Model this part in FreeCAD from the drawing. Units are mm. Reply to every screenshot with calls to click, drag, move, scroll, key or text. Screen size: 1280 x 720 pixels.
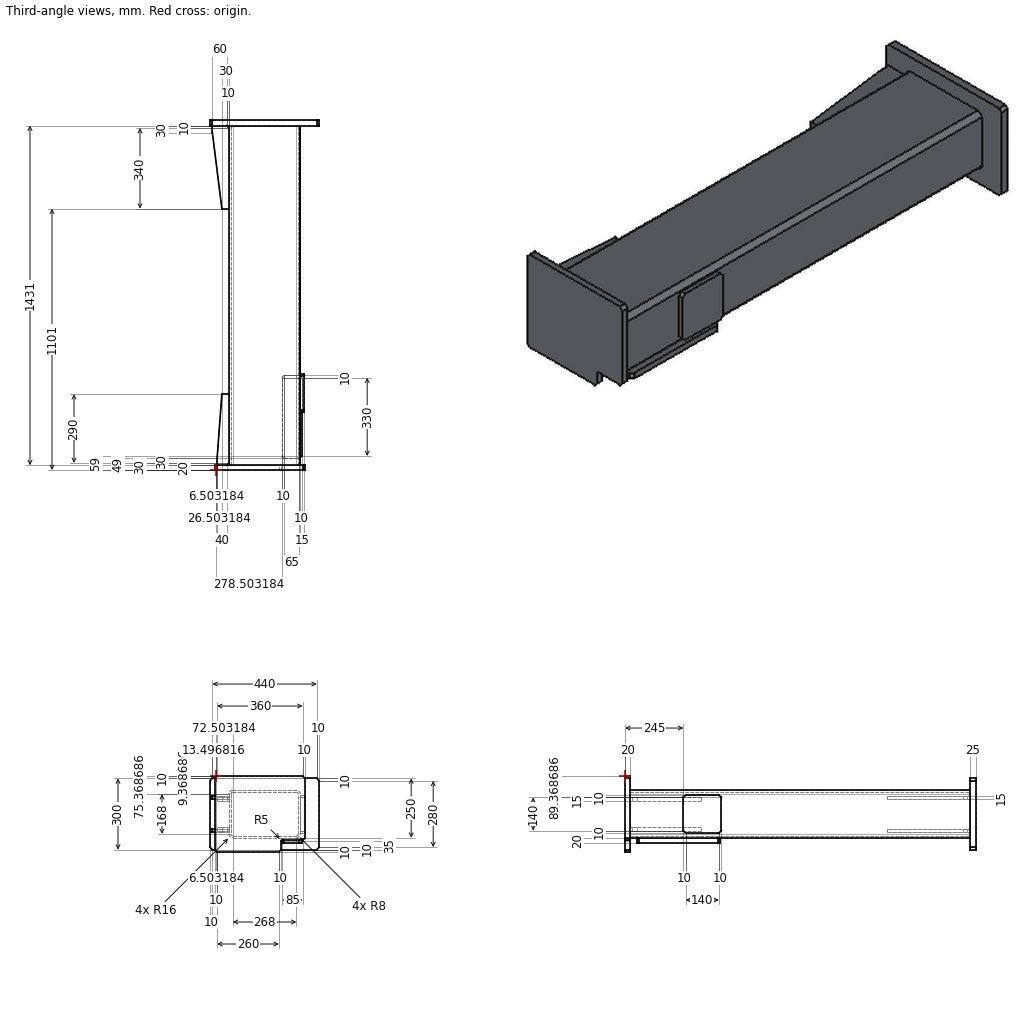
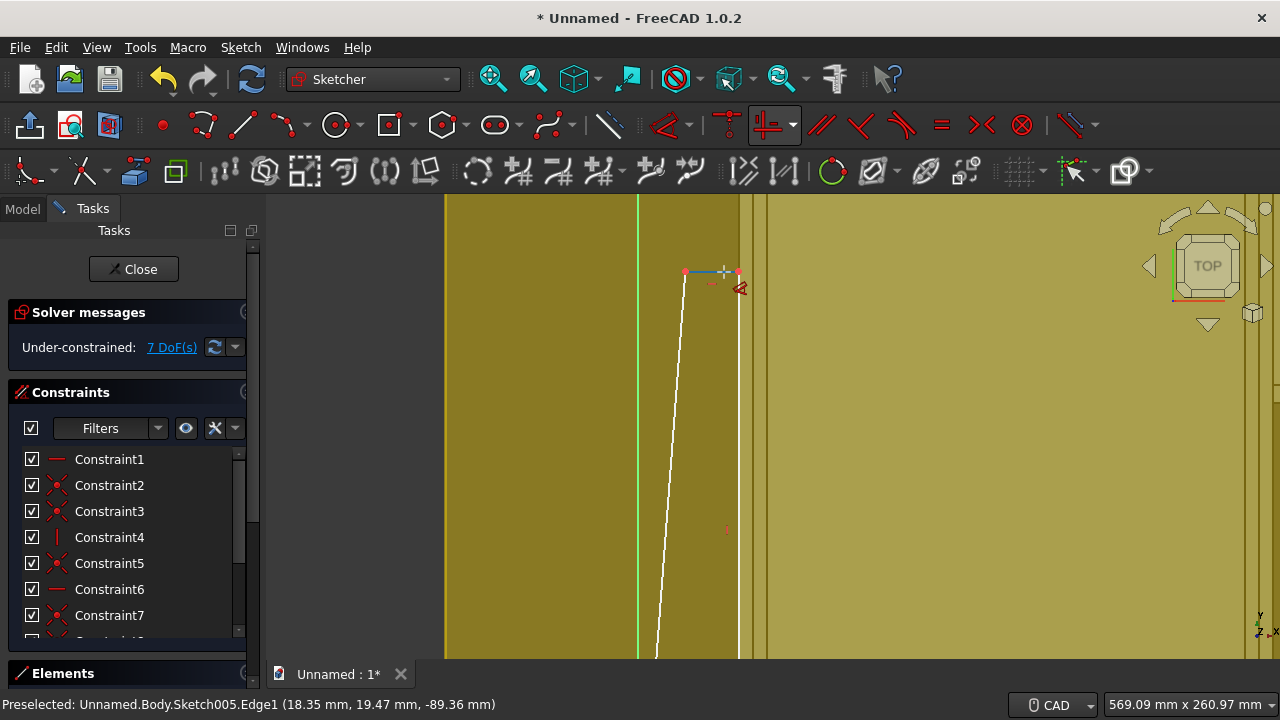
click(723, 272)
click(712, 238)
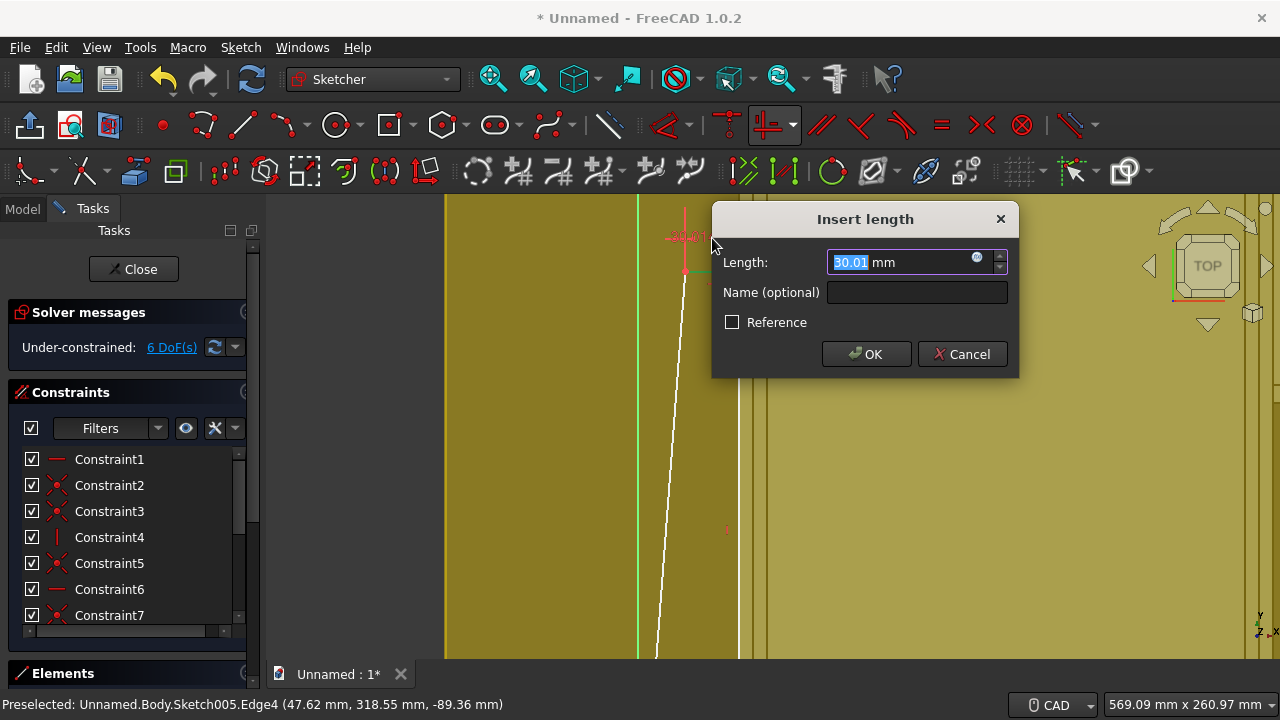
text(30)
key(Return)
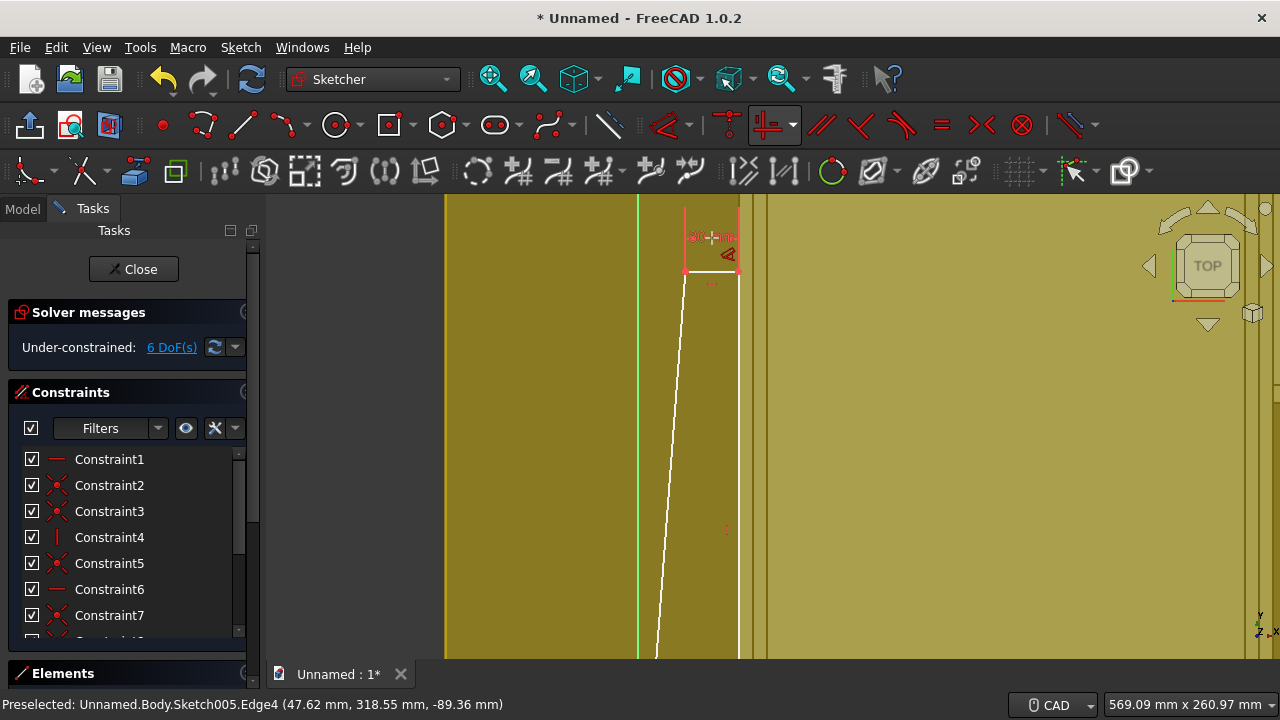
scroll(724, 271, down, 3)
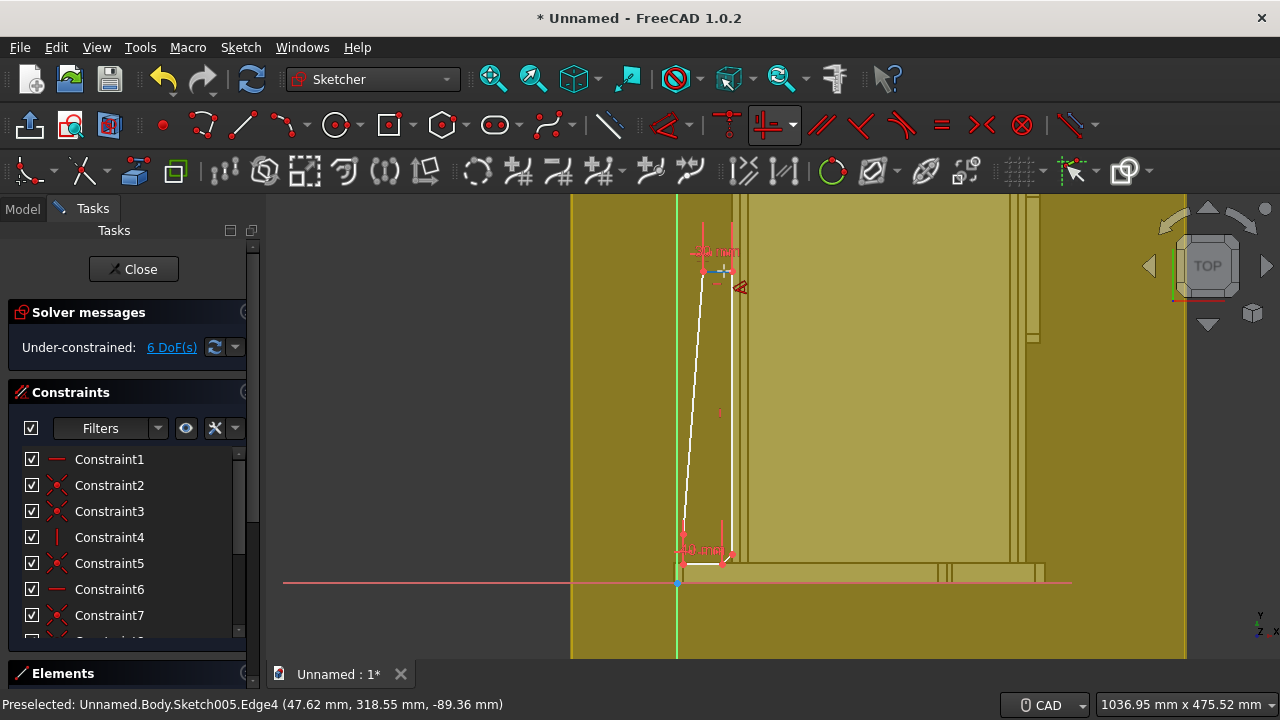
scroll(683, 543, up, 5)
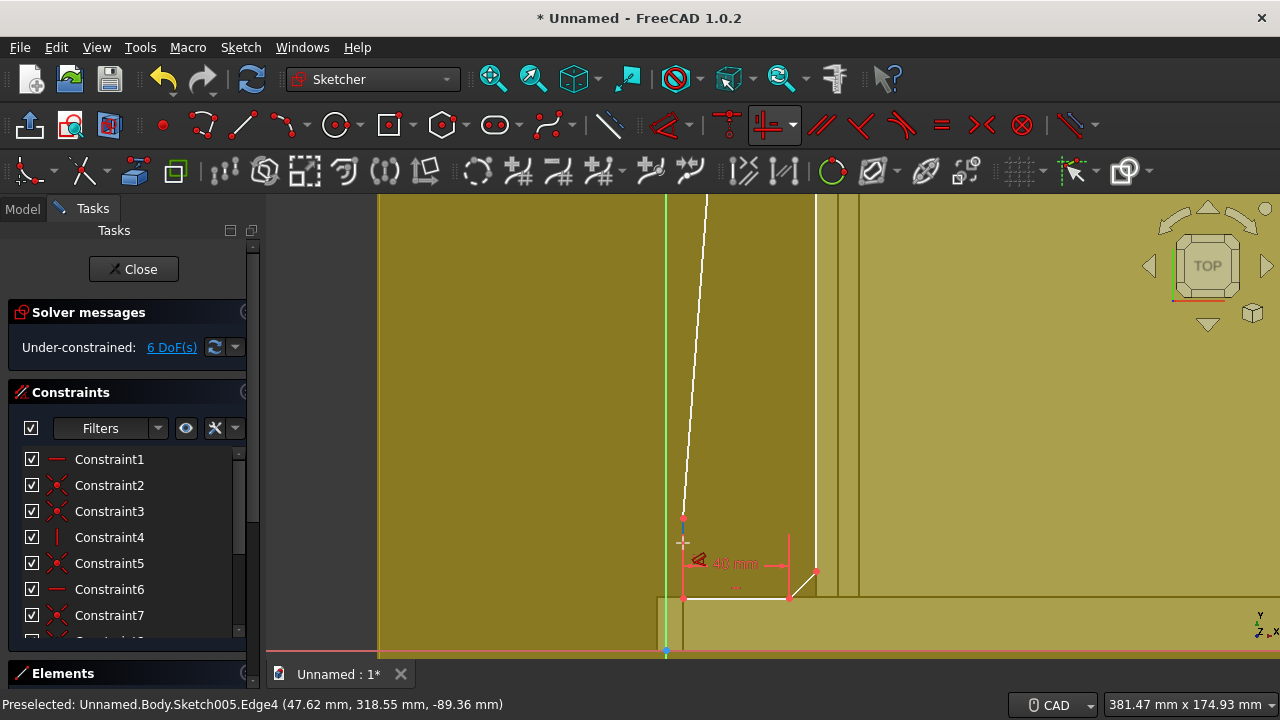
click(683, 543)
click(649, 559)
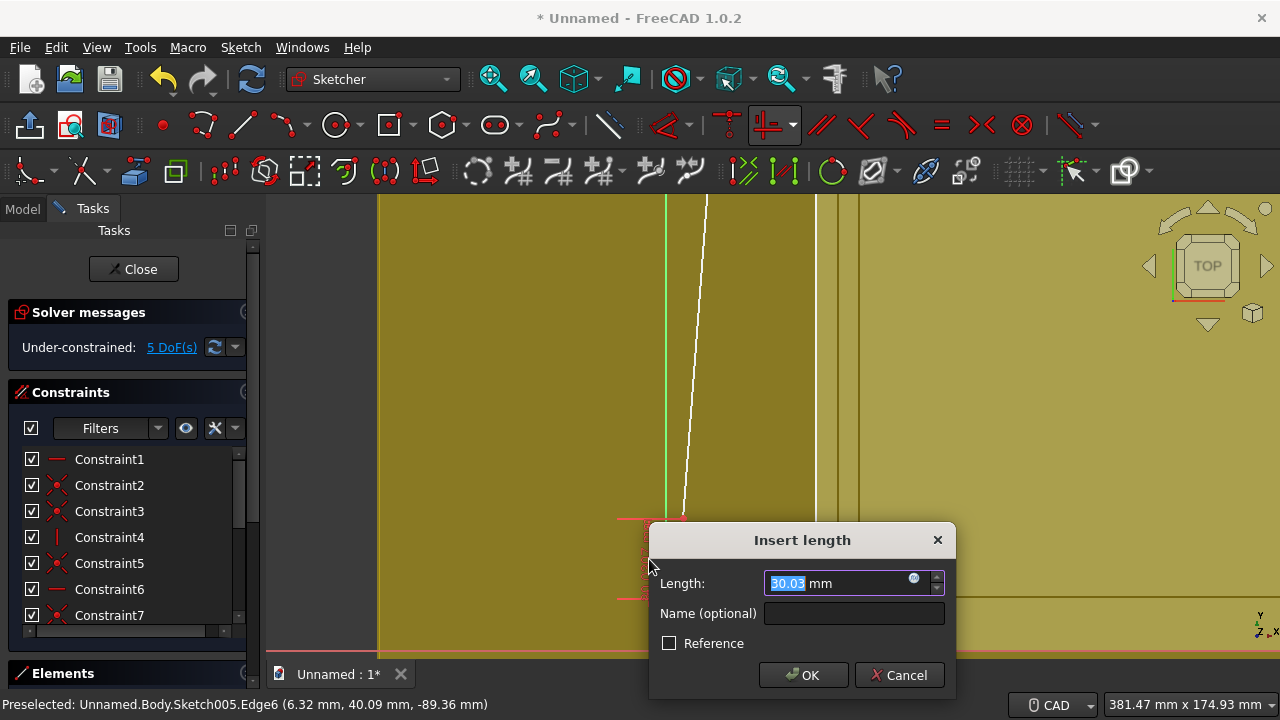
text(30)
key(Return)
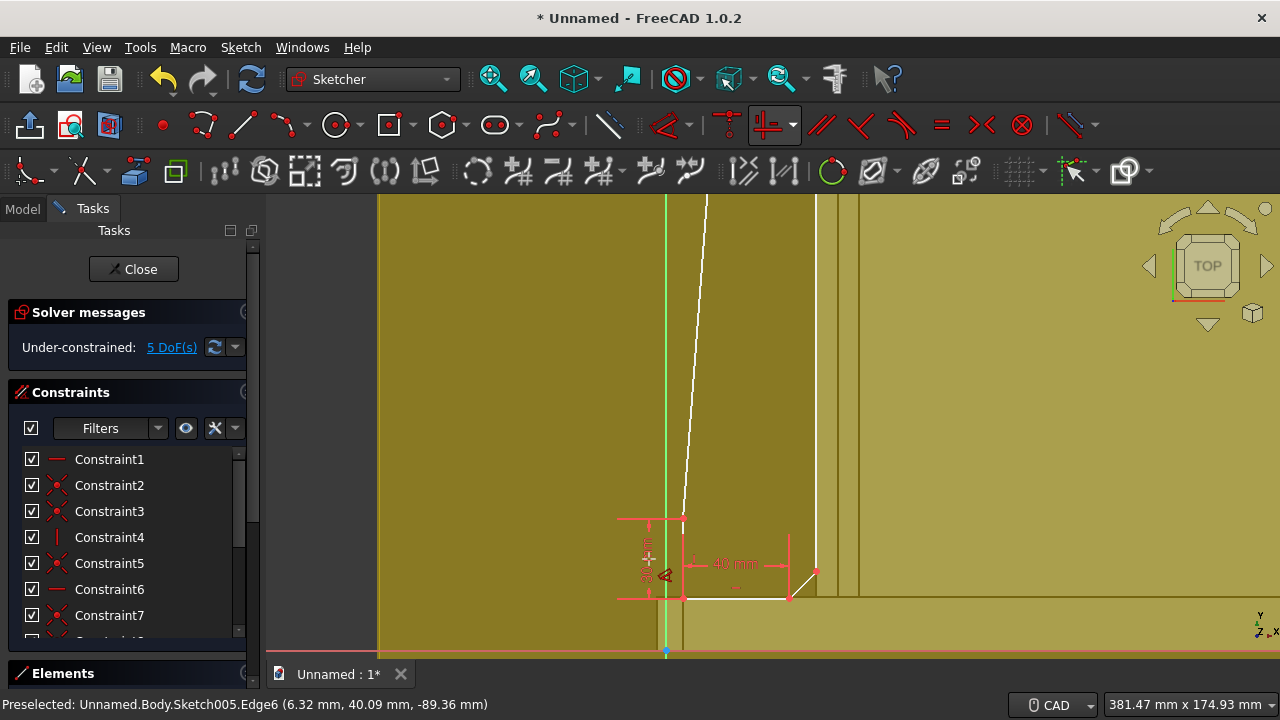
click(816, 341)
click(850, 397)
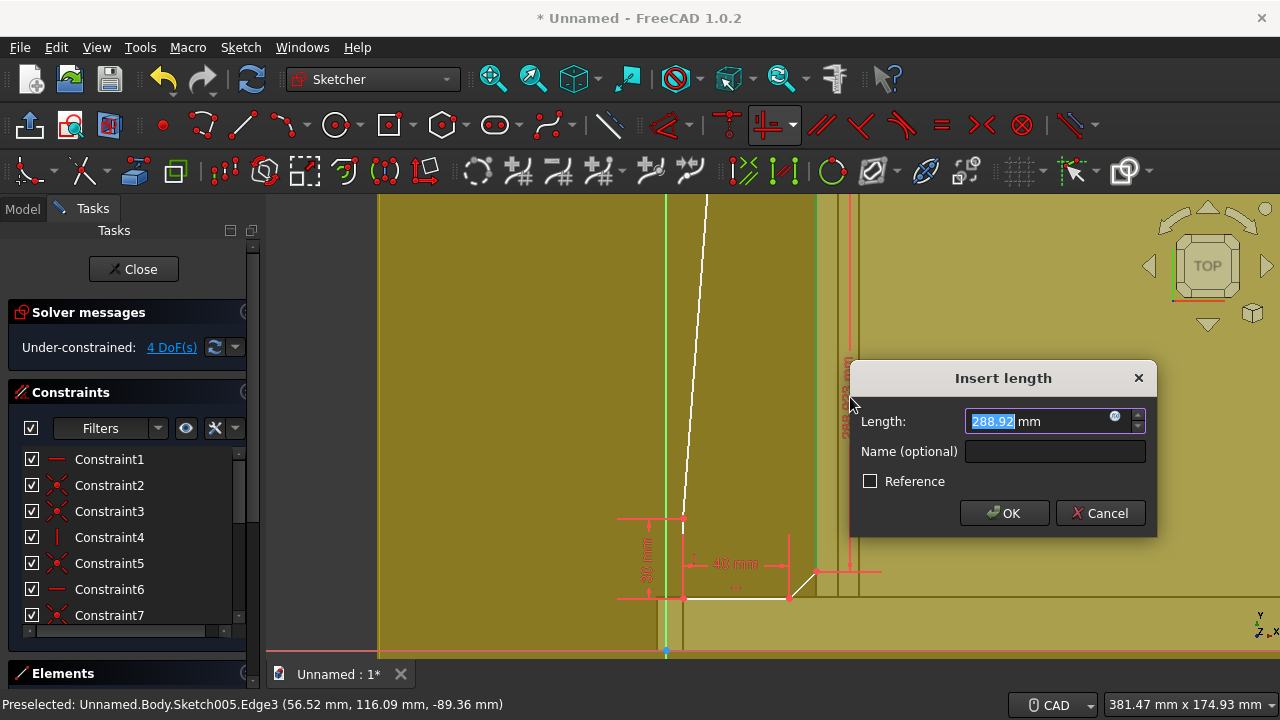
text(290)
key(Return)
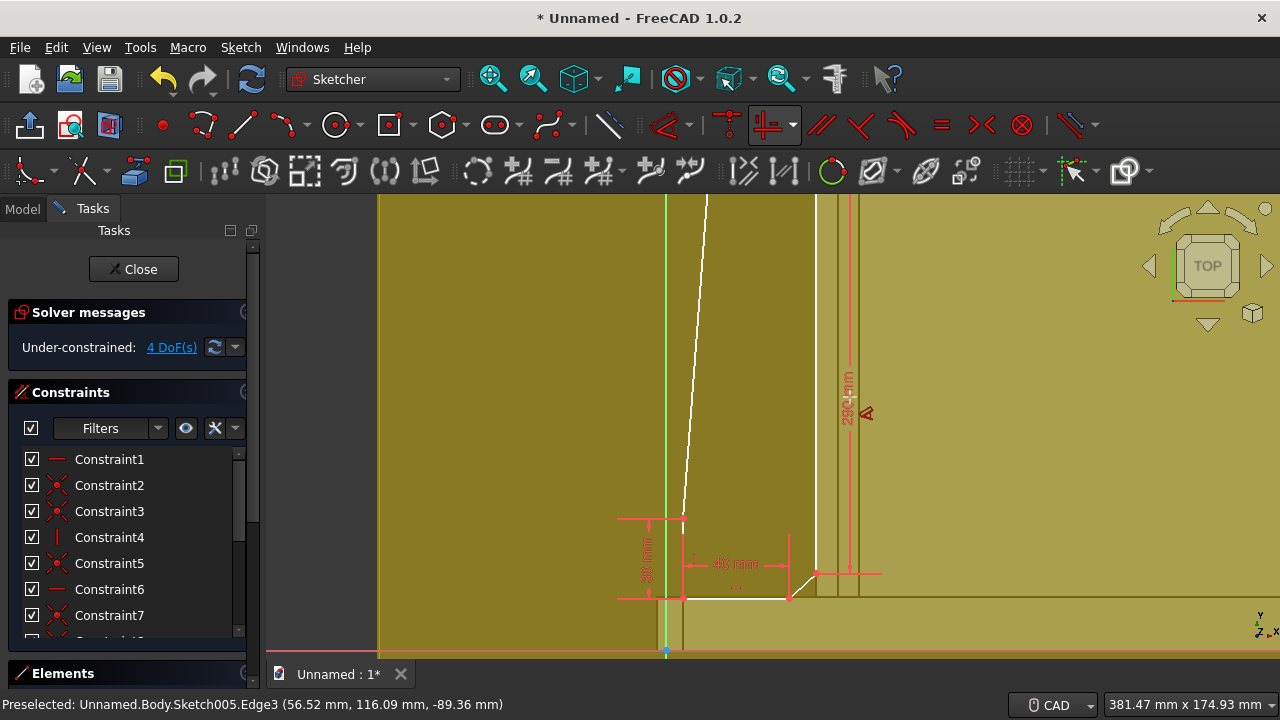
click(683, 599)
click(632, 615)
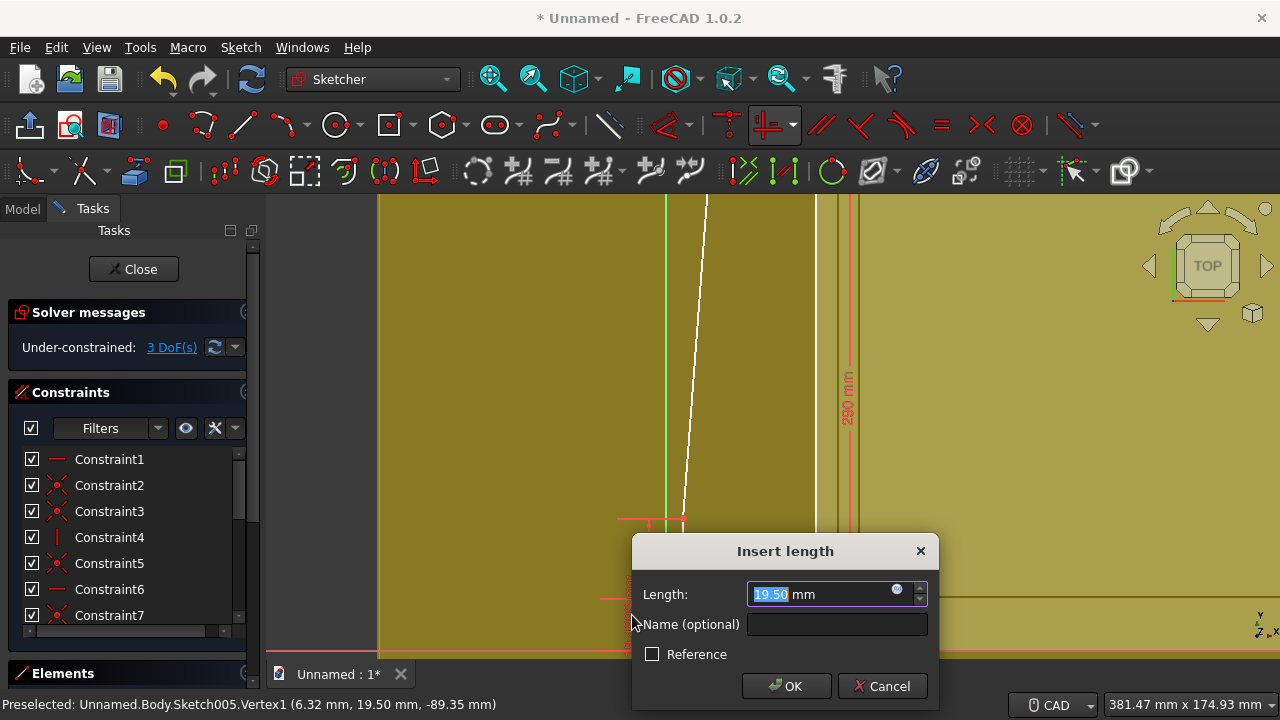
text(20)
key(Return)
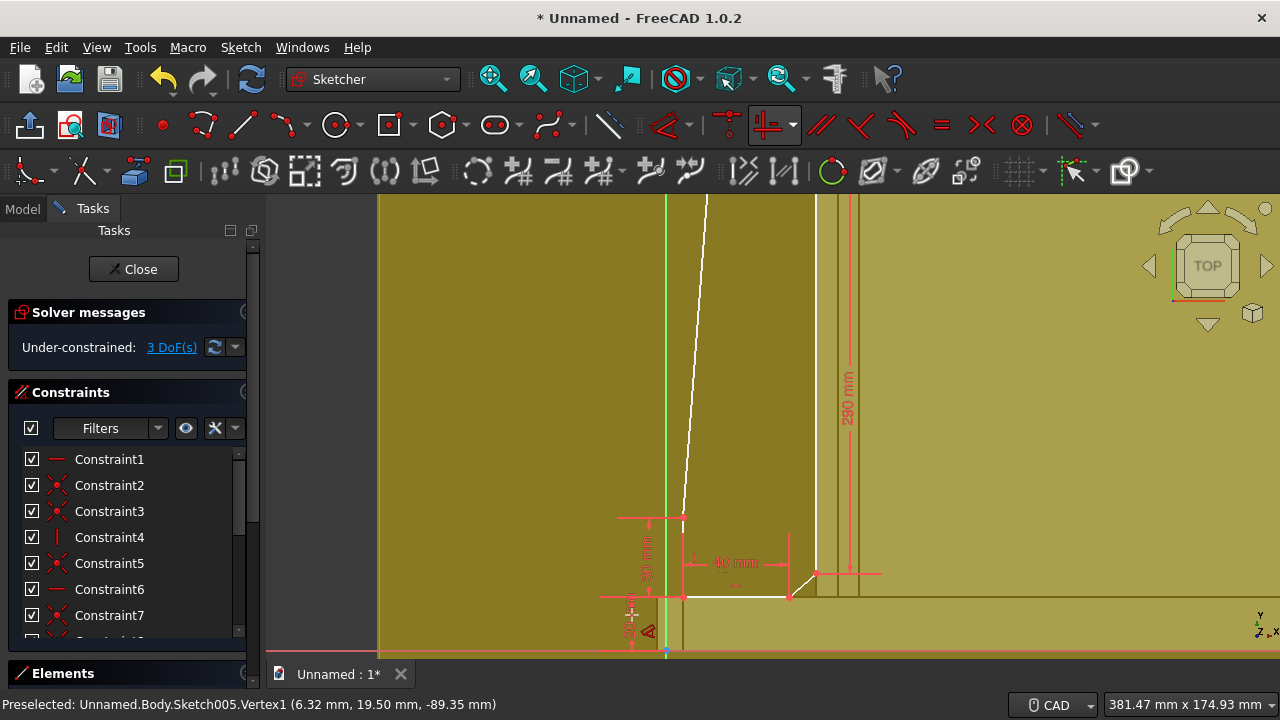
click(816, 574)
click(850, 602)